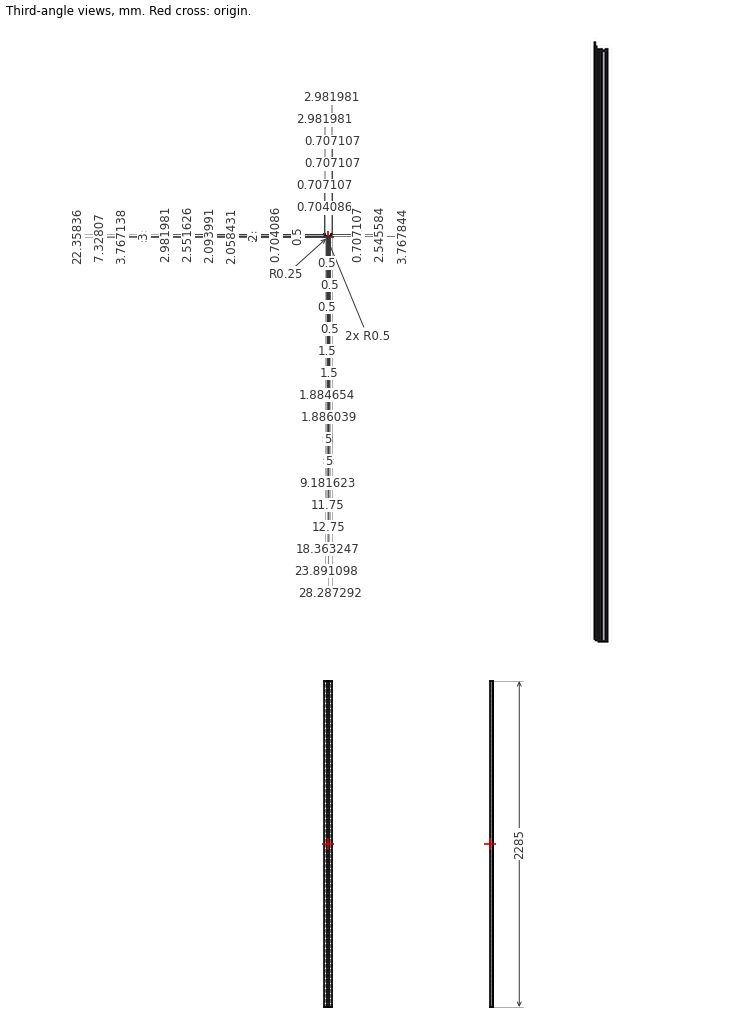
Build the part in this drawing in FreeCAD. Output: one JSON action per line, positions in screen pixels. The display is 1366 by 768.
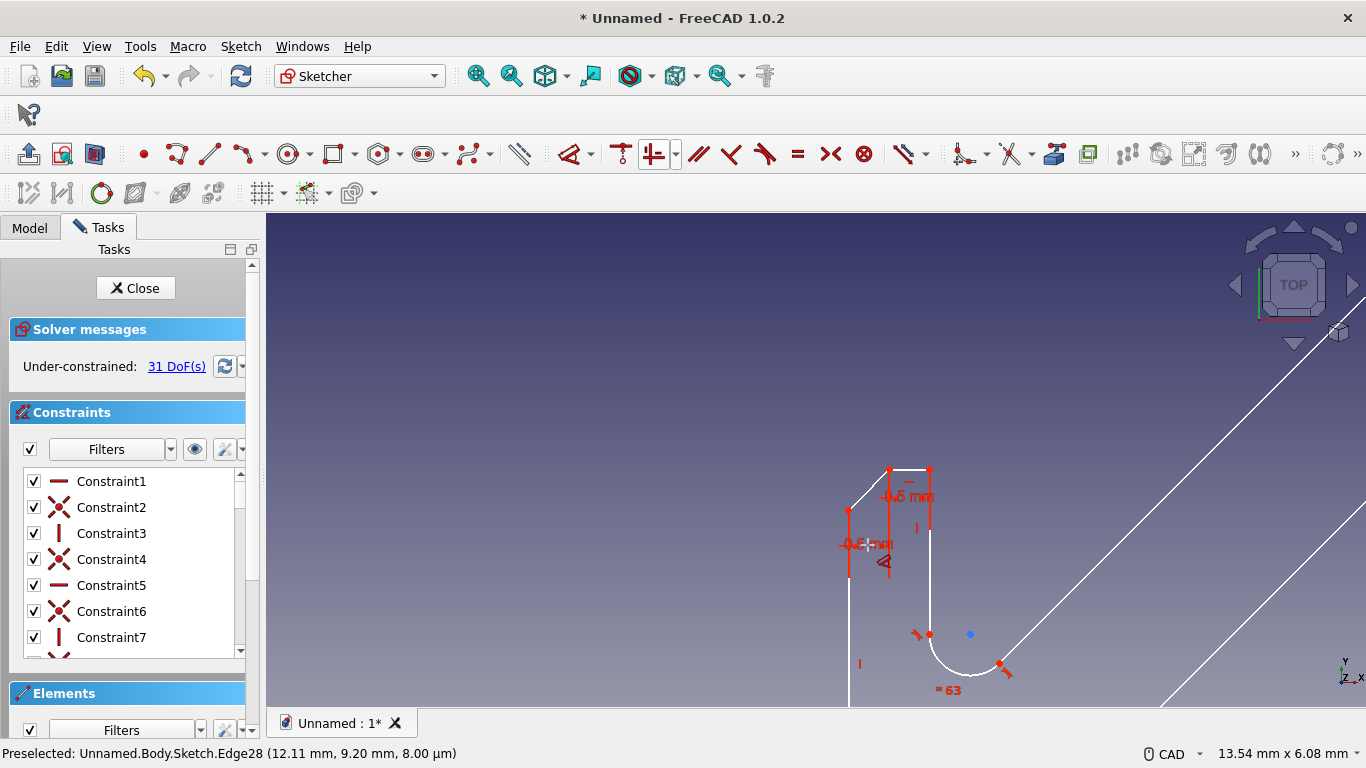
{"action": "left_click", "coordinate": [877, 482]}
{"action": "left_click", "coordinate": [815, 490]}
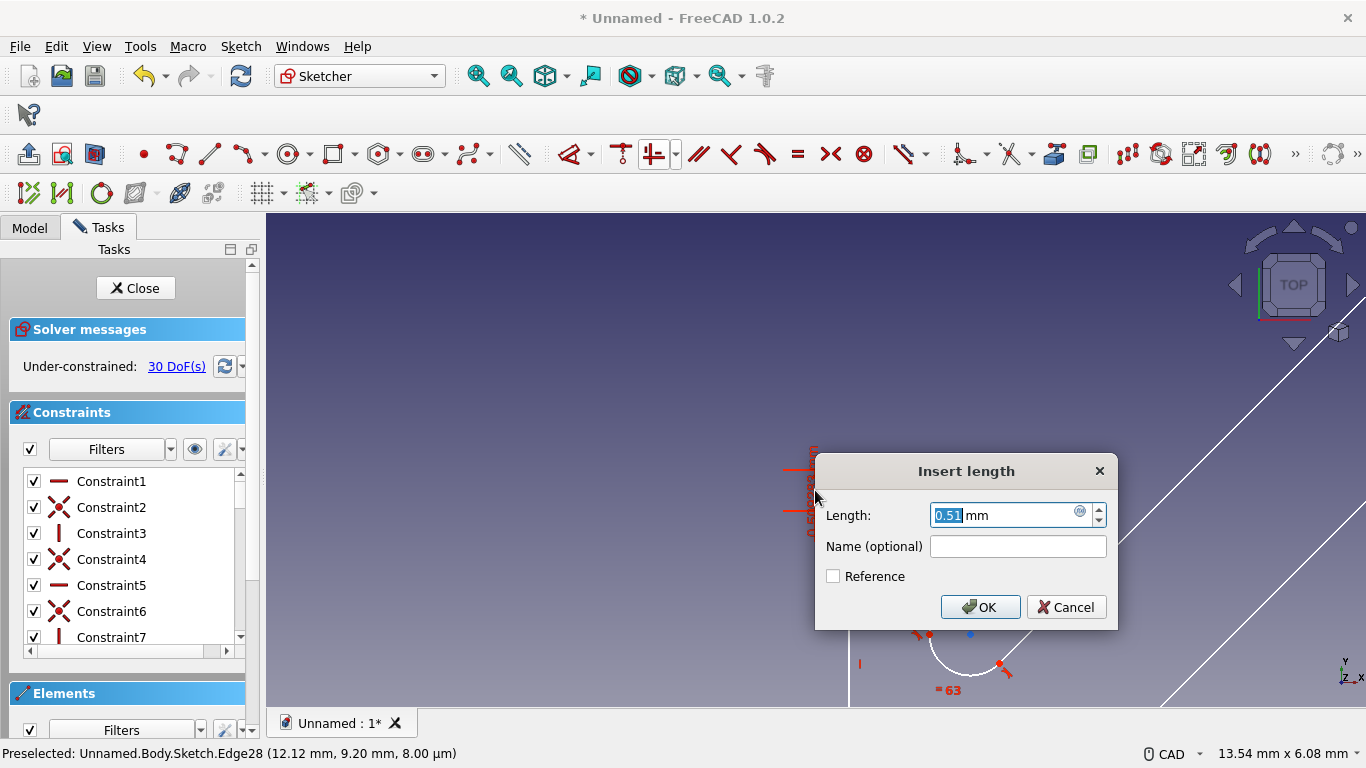
{"action": "type", "text": "0.5"}
{"action": "key", "text": "Return"}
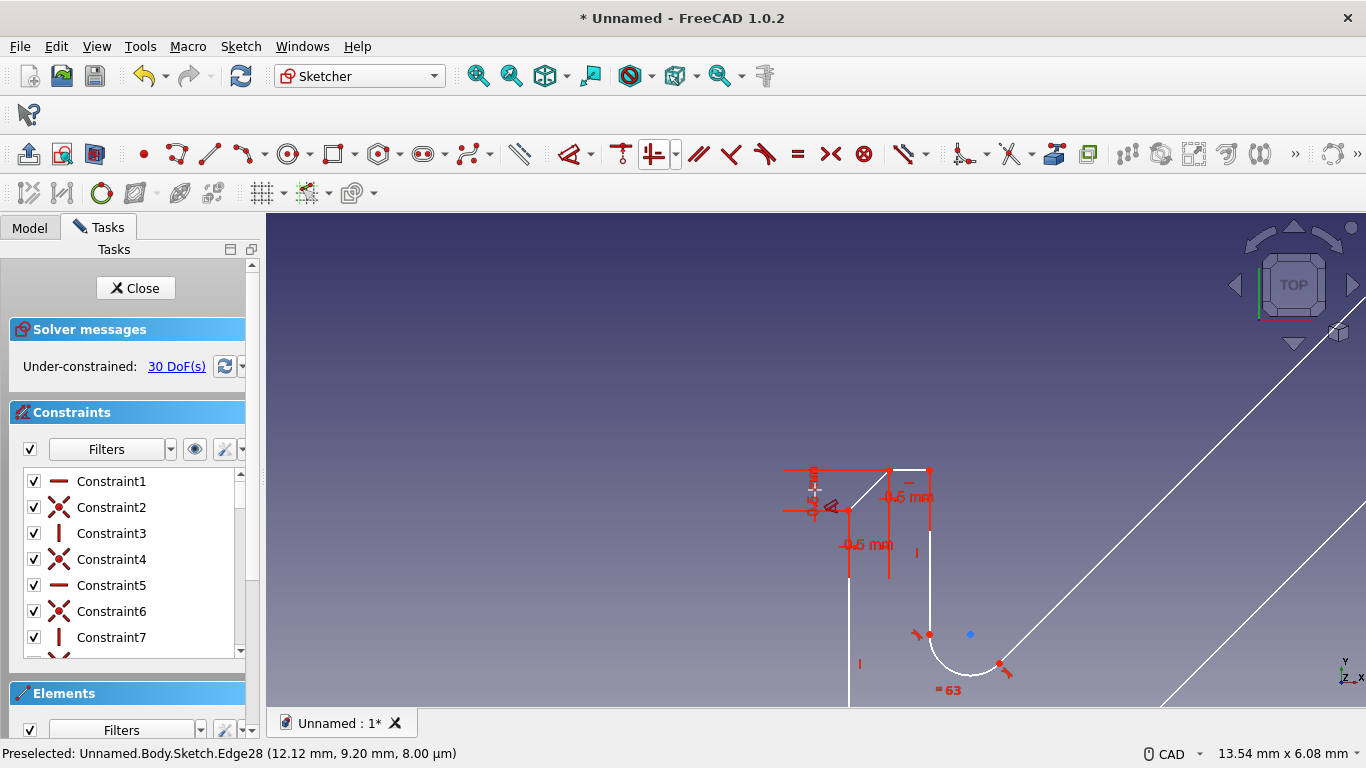
{"action": "scroll", "coordinate": [881, 482], "scroll_direction": "down", "scroll_amount": 10}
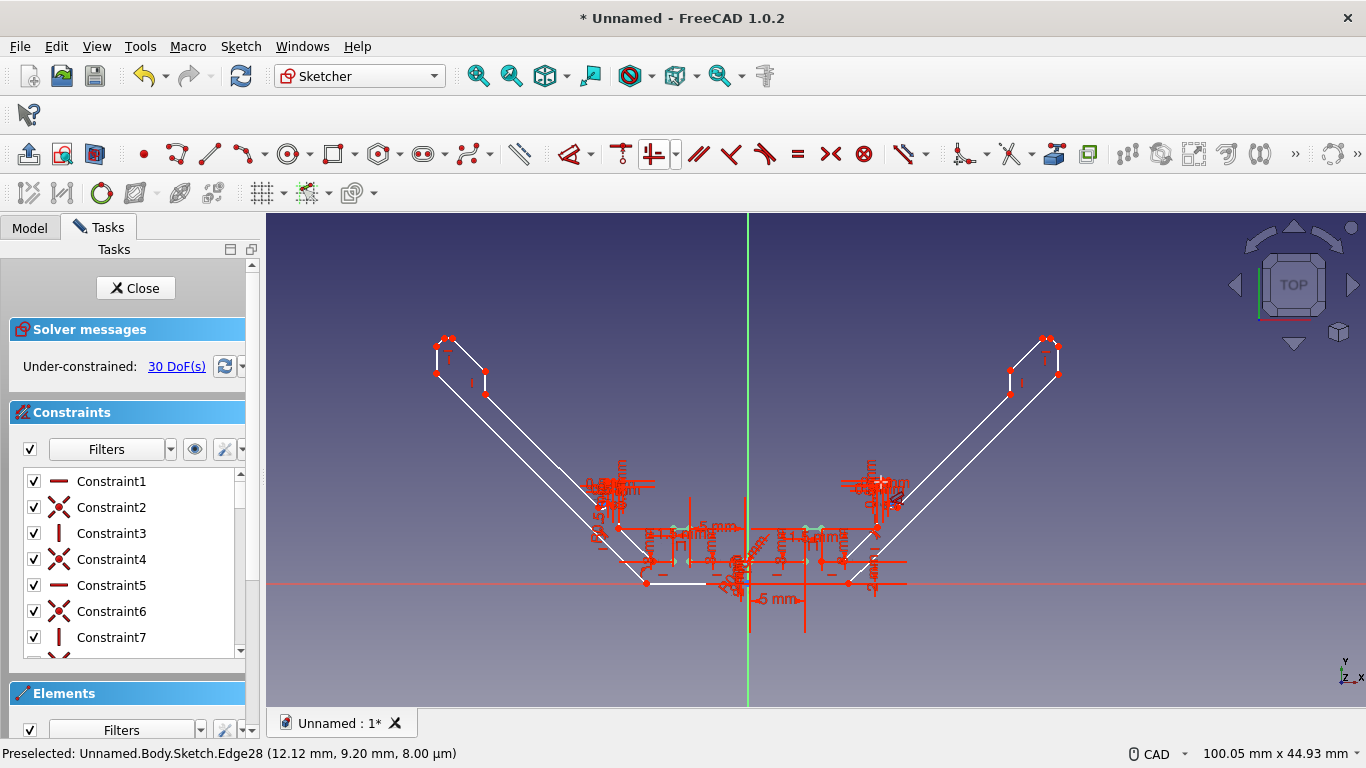
{"action": "left_click", "coordinate": [619, 529]}
{"action": "left_click", "coordinate": [683, 618]}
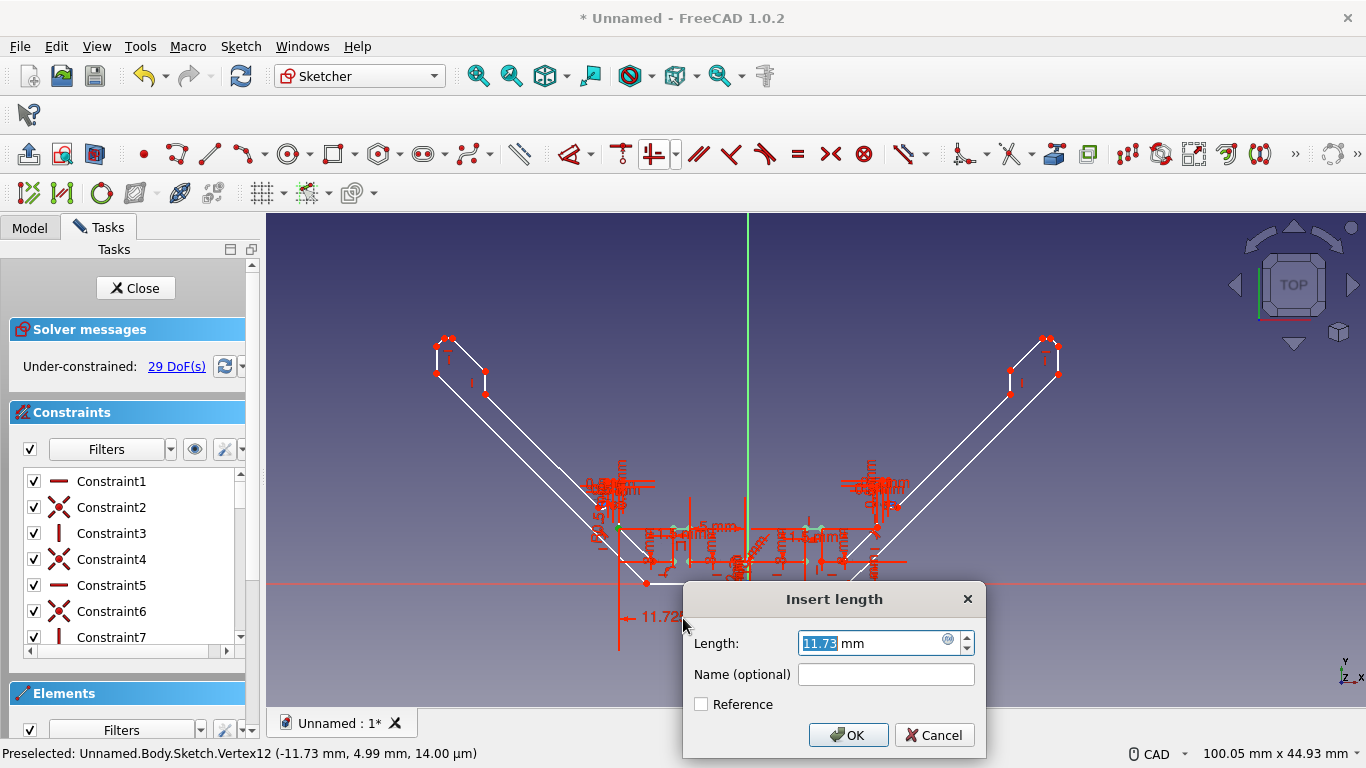
{"action": "type", "text": "11.75"}
{"action": "key", "text": "Return"}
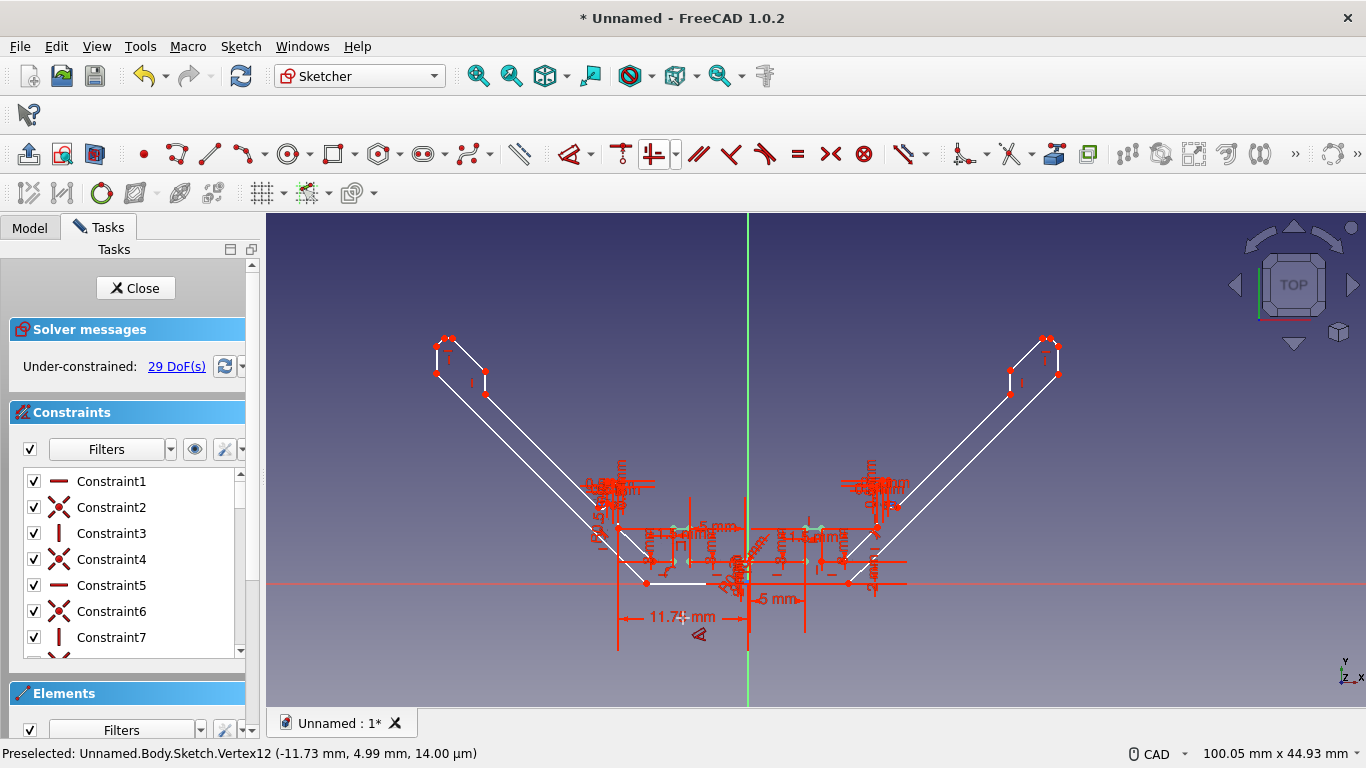
{"action": "scroll", "coordinate": [888, 503], "scroll_direction": "up", "scroll_amount": 4}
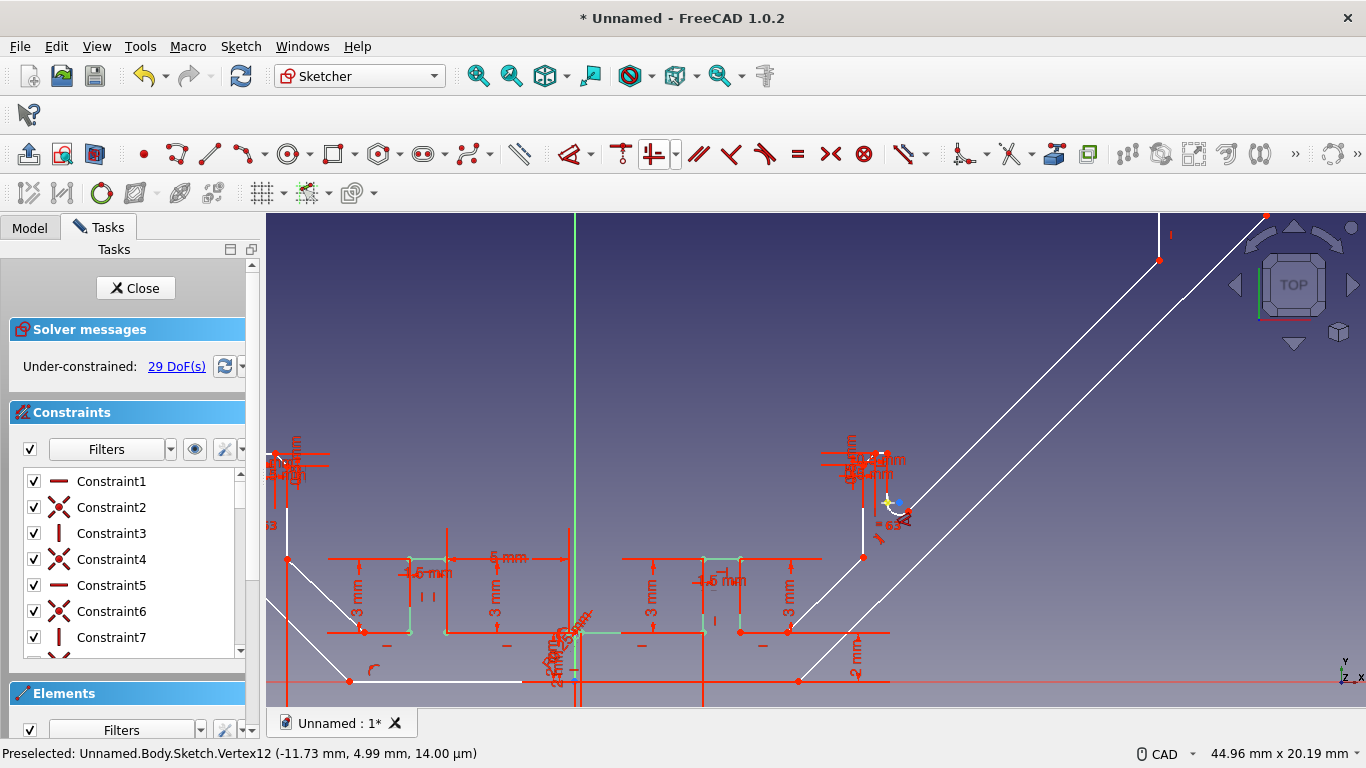
{"action": "left_click", "coordinate": [887, 503]}
{"action": "left_click", "coordinate": [731, 469]}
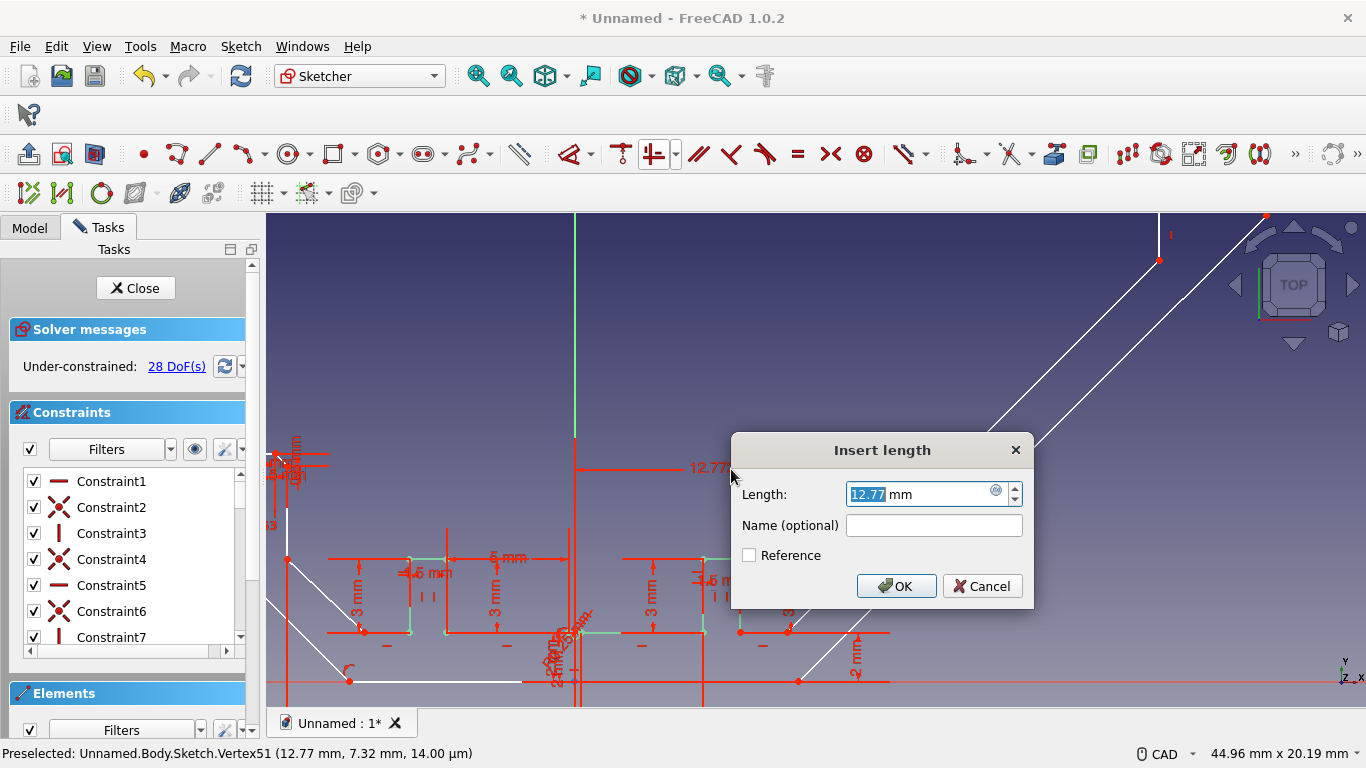
{"action": "type", "text": "12.75"}
{"action": "key", "text": "Return"}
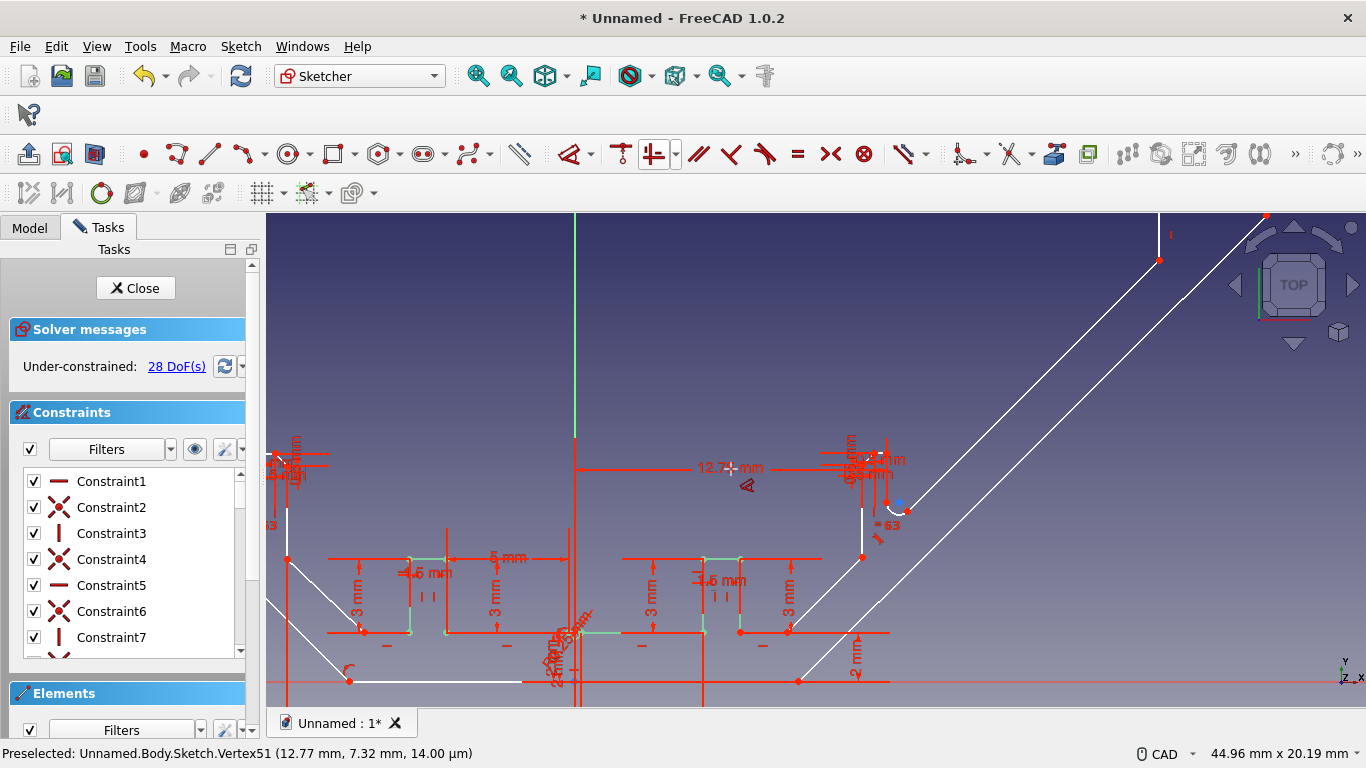
{"action": "left_click", "coordinate": [396, 633]}
{"action": "left_click", "coordinate": [387, 667]}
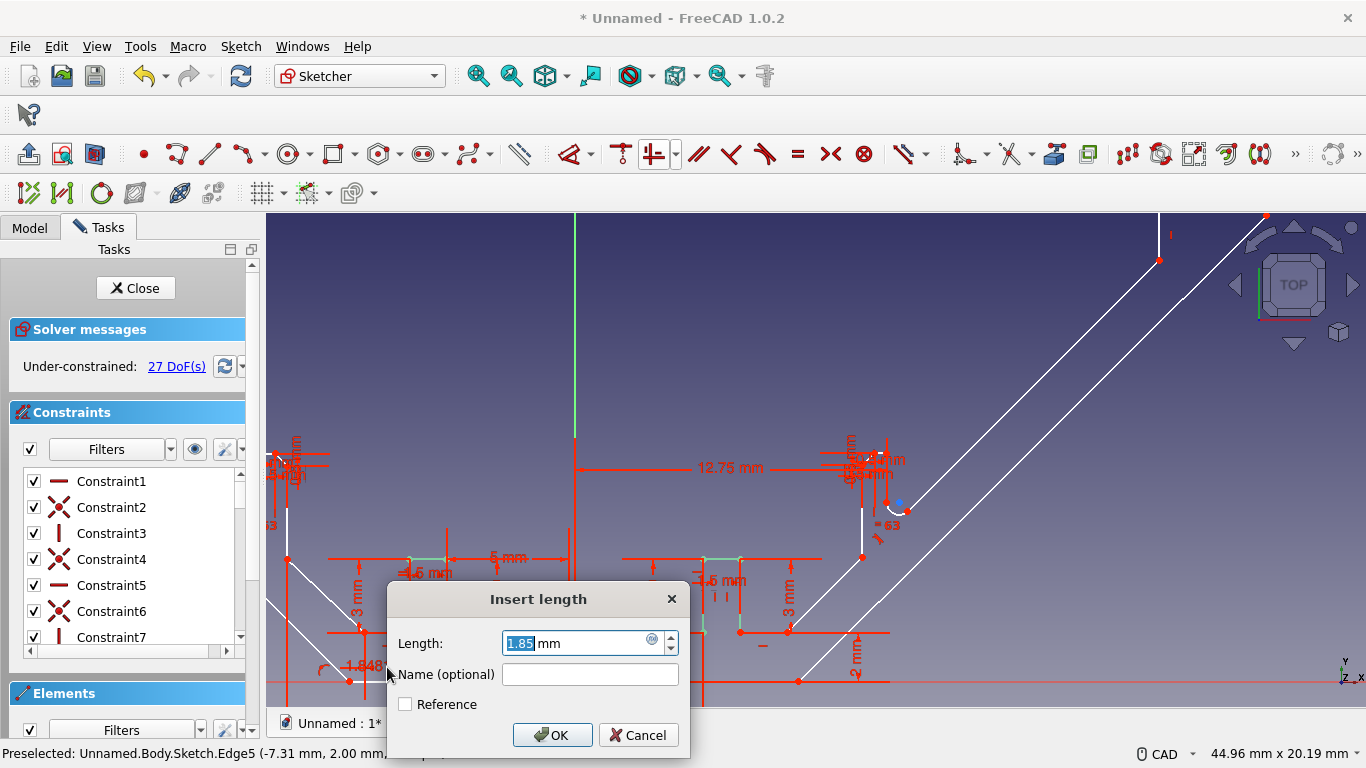
{"action": "type", "text": "1.884654"}
{"action": "key", "text": "Return"}